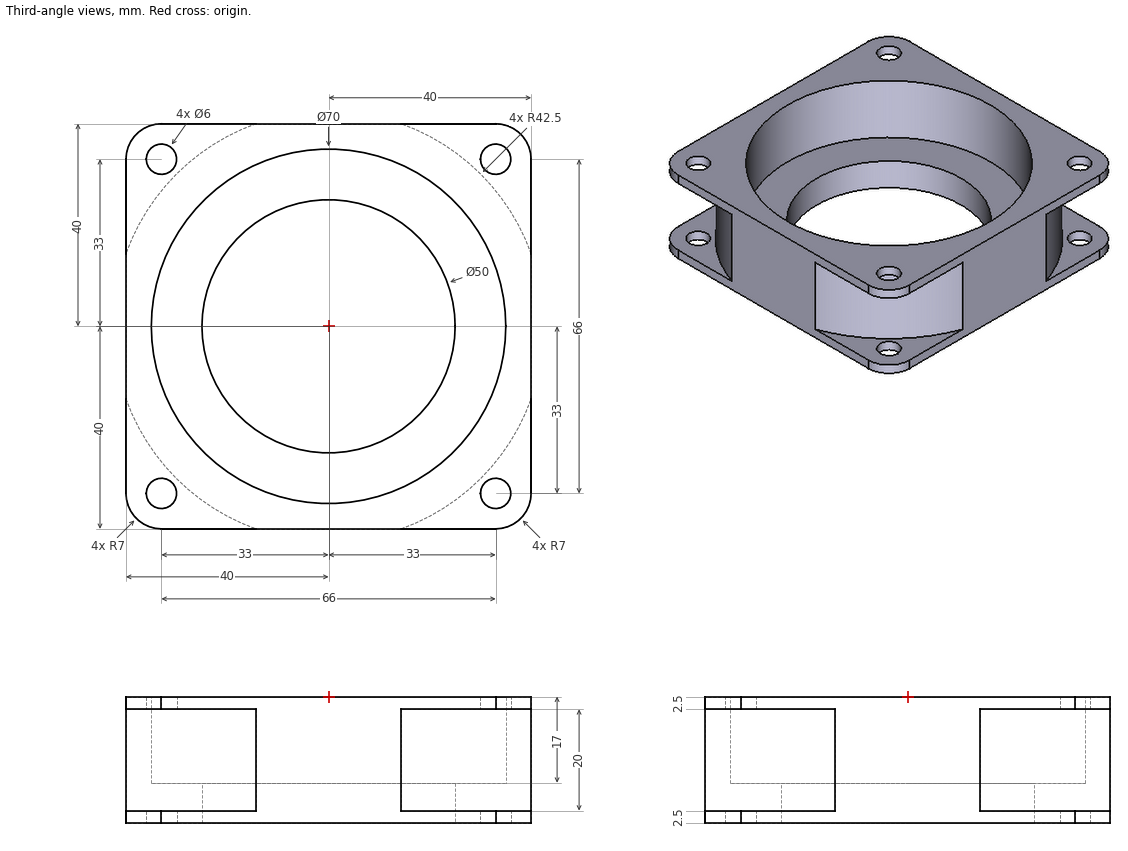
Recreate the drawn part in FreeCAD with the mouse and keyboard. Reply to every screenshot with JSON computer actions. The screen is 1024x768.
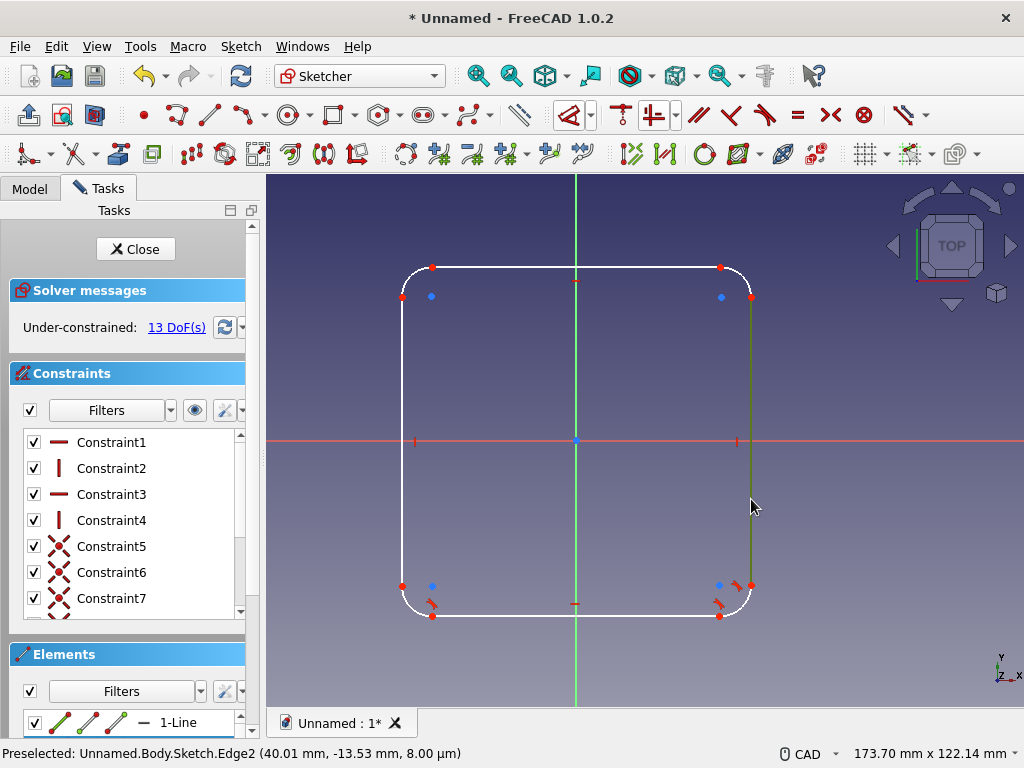
{"action": "left_click", "coordinate": [748, 284]}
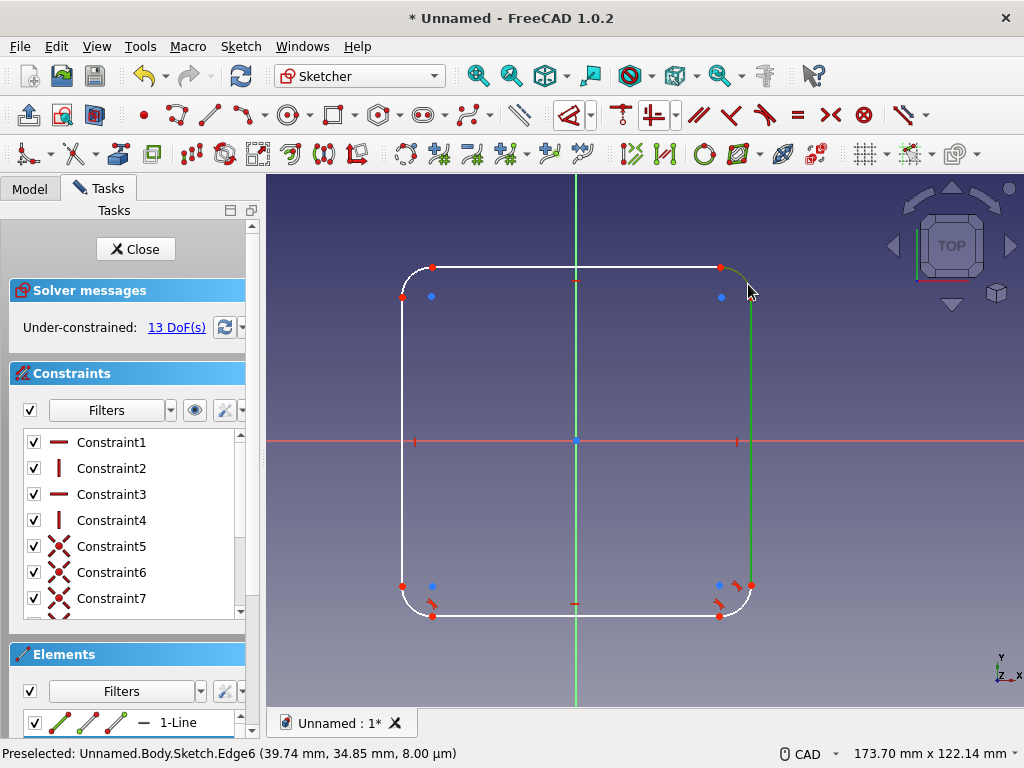
{"action": "left_click", "coordinate": [765, 116]}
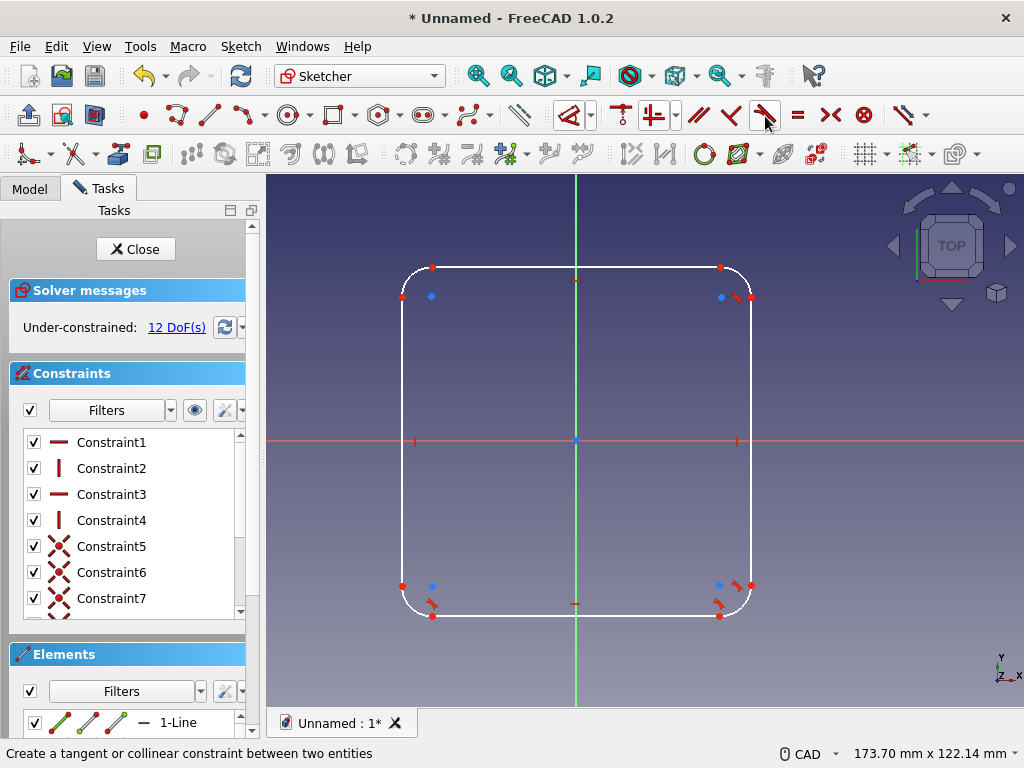
{"action": "left_click", "coordinate": [634, 267]}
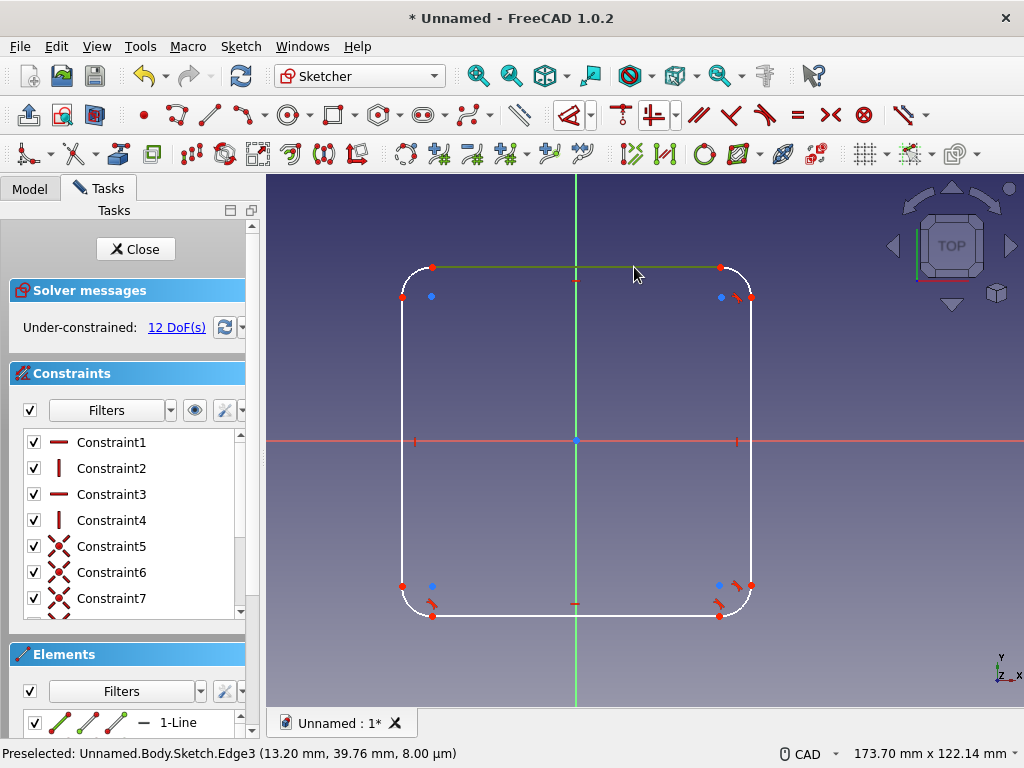
{"action": "left_click", "coordinate": [748, 284]}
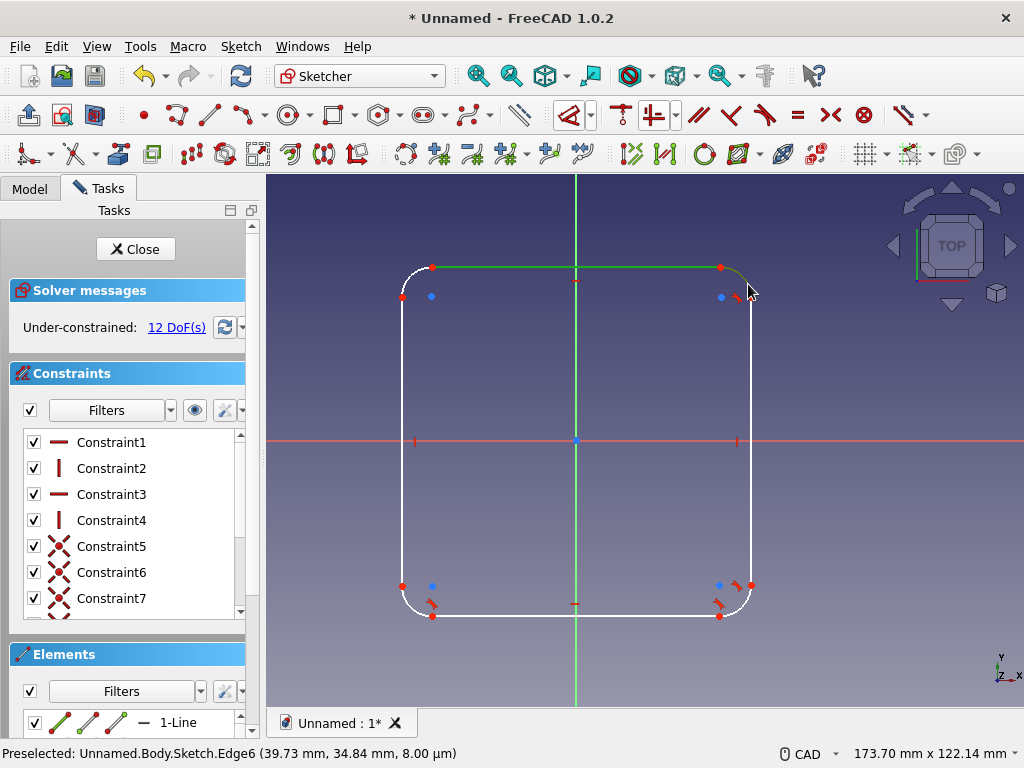
{"action": "left_click", "coordinate": [765, 116]}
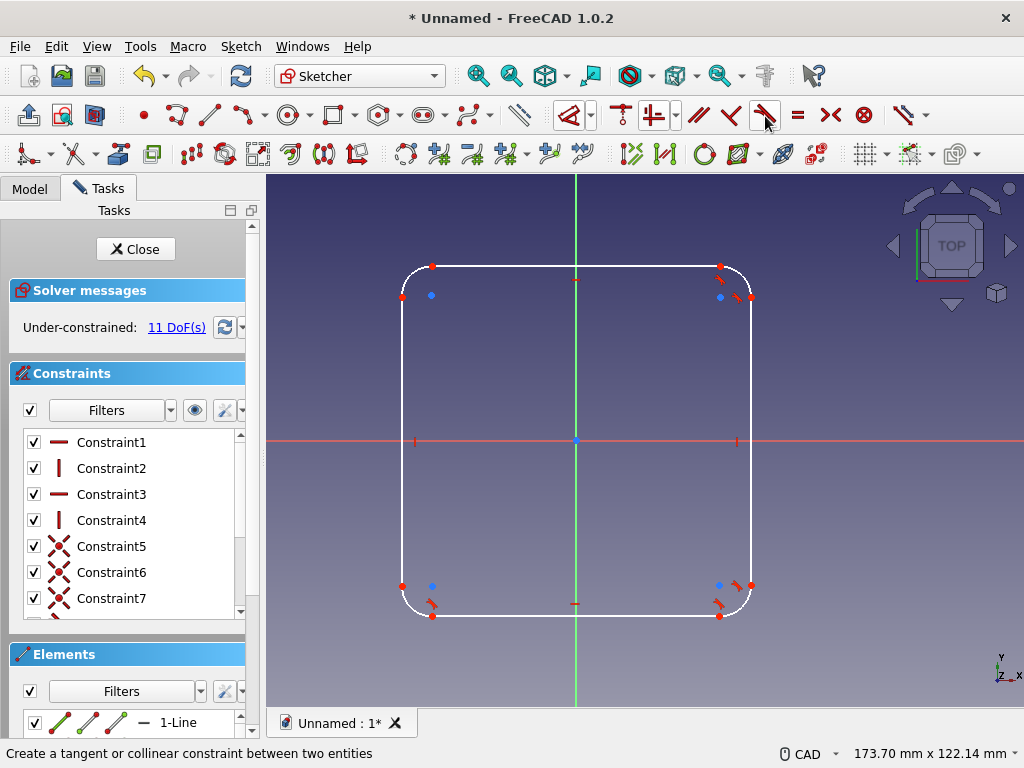
{"action": "left_click", "coordinate": [634, 266]}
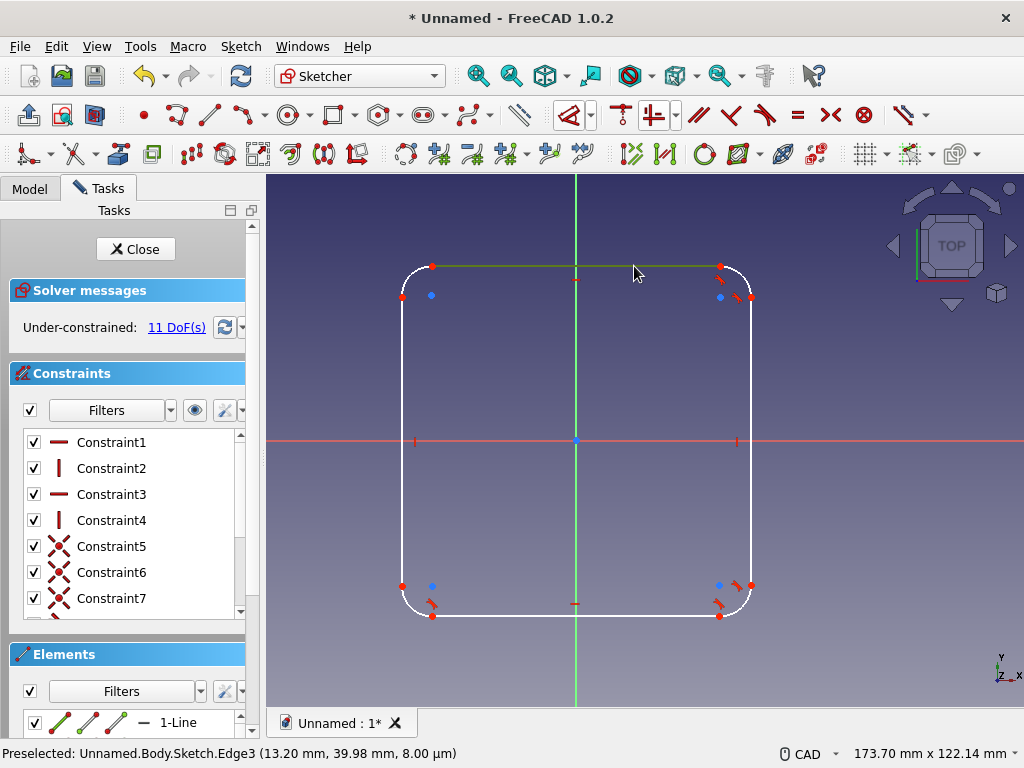
{"action": "left_click", "coordinate": [418, 270]}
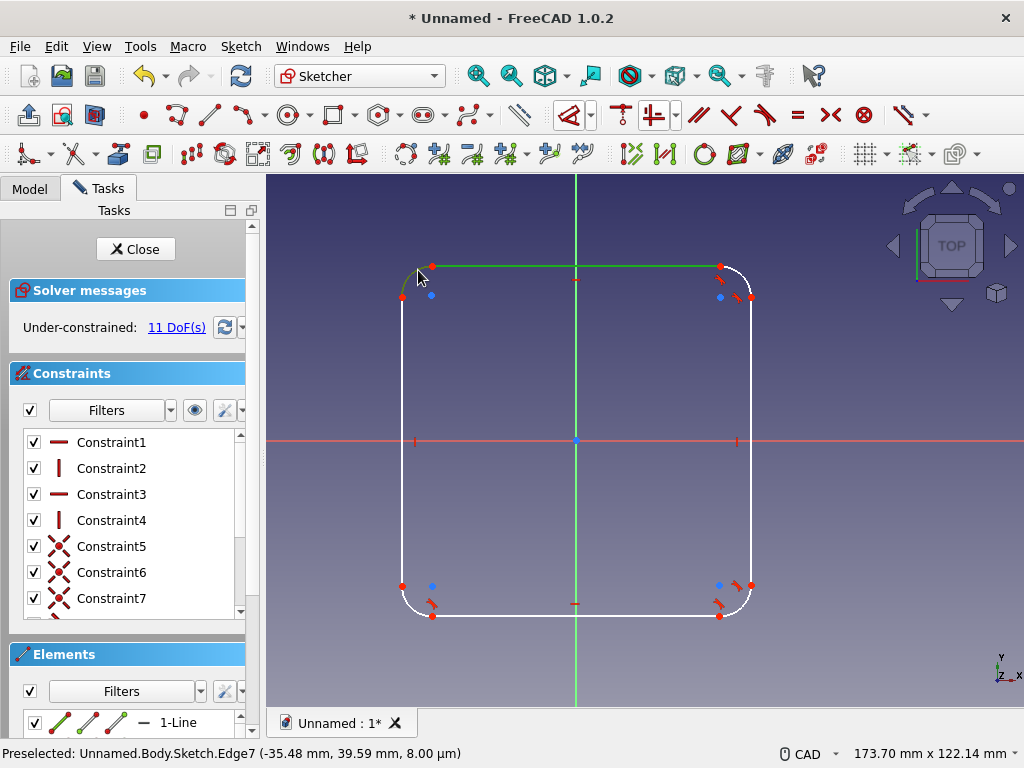
{"action": "left_click", "coordinate": [765, 116]}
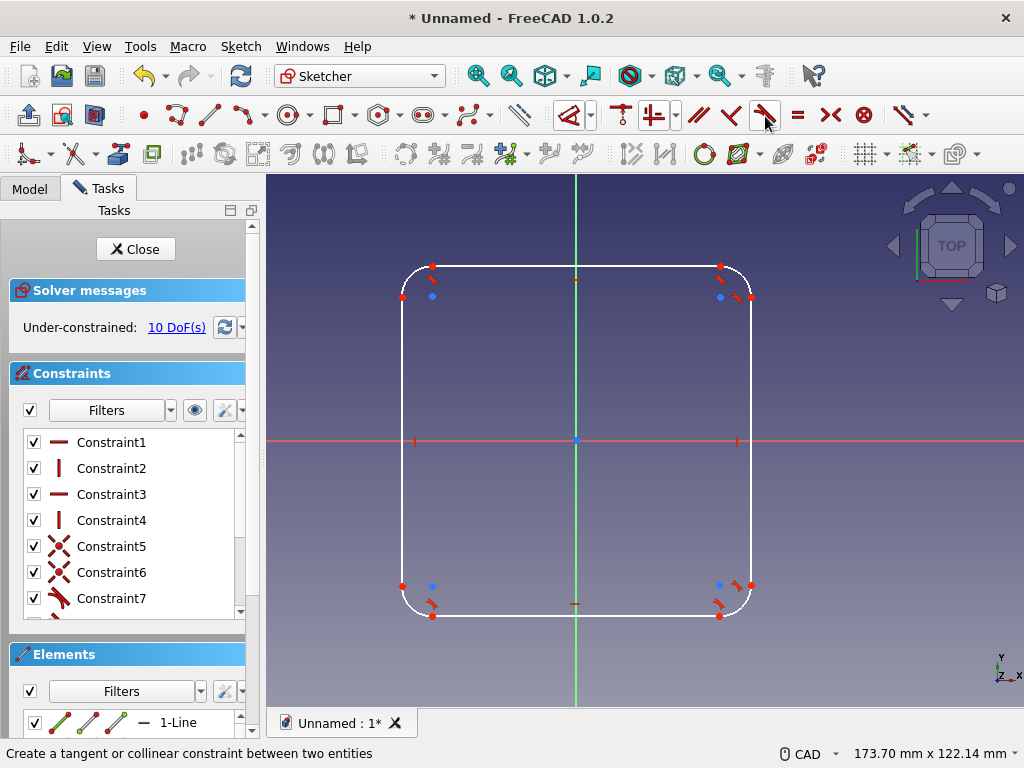
{"action": "left_click", "coordinate": [402, 384]}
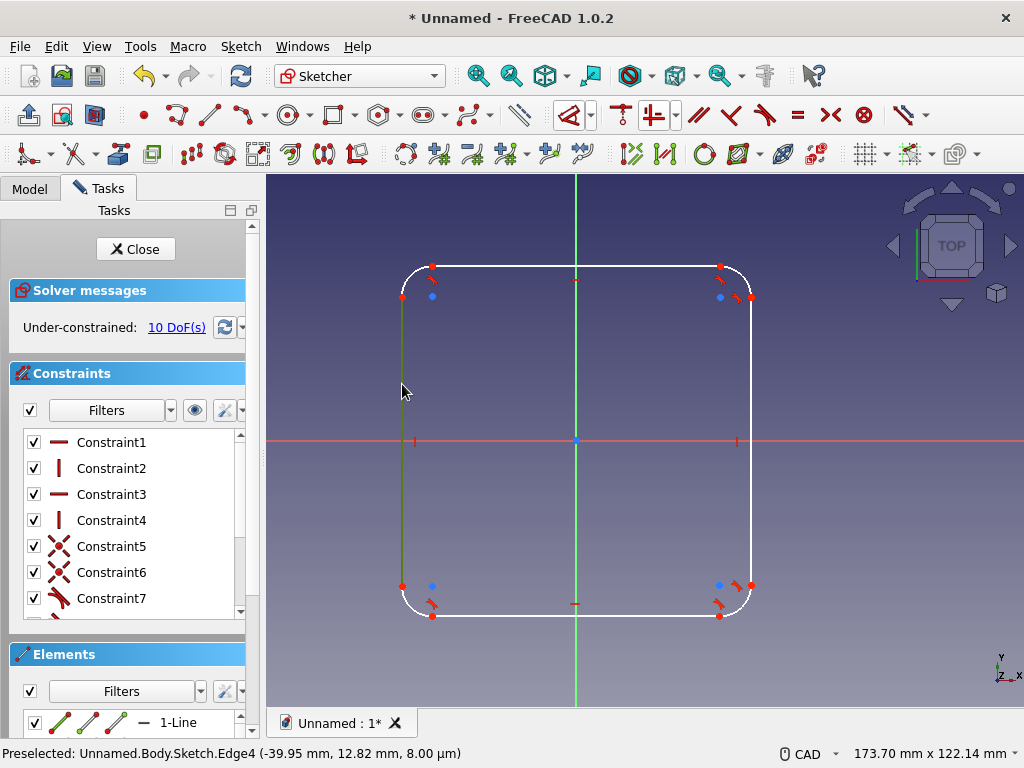
{"action": "left_click", "coordinate": [418, 270]}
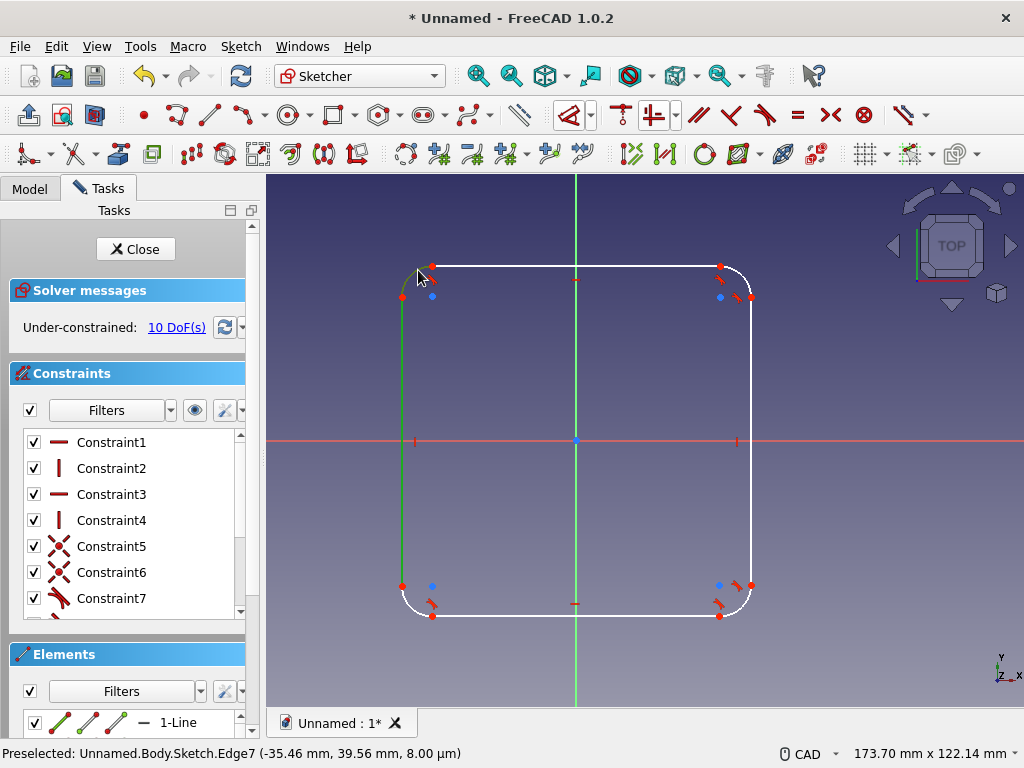
{"action": "left_click", "coordinate": [765, 116]}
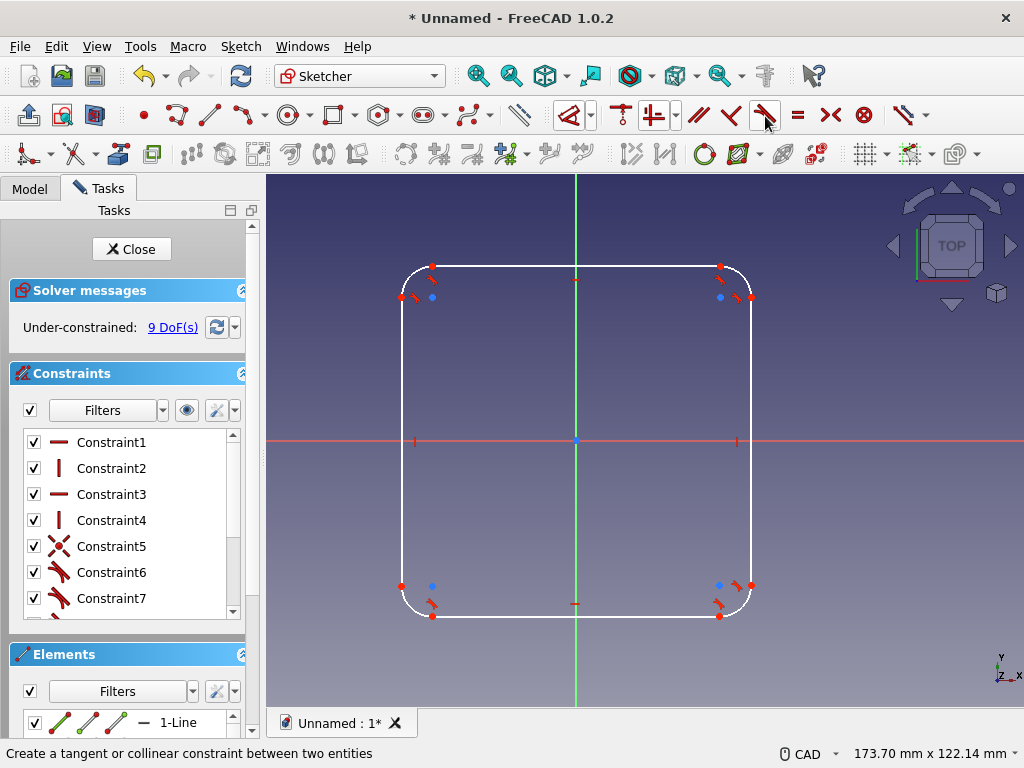
{"action": "left_click", "coordinate": [402, 384]}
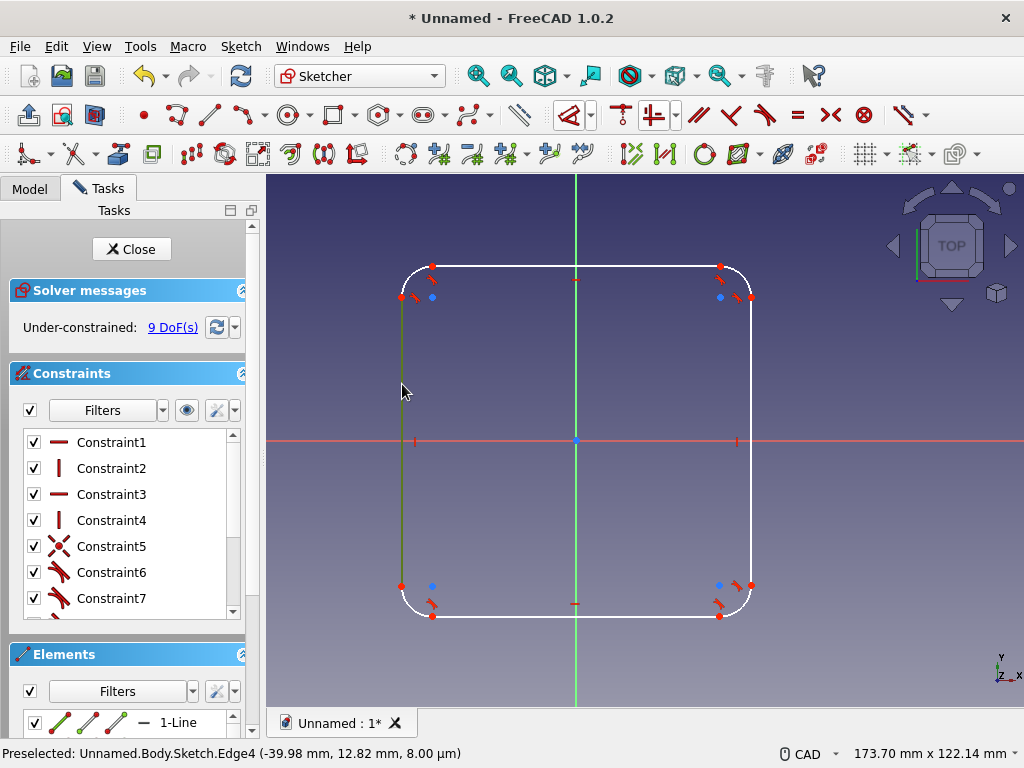
{"action": "left_click", "coordinate": [405, 600]}